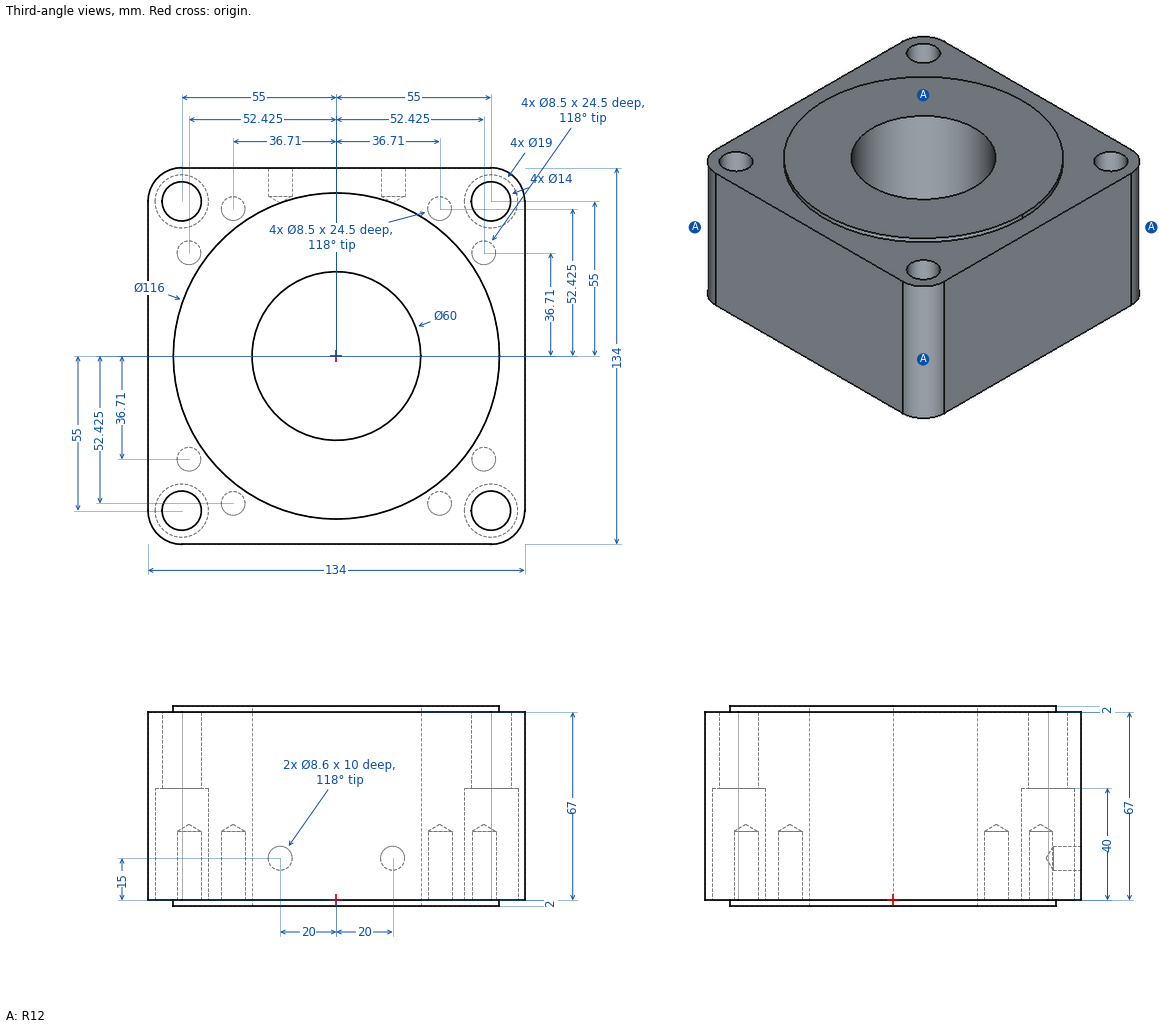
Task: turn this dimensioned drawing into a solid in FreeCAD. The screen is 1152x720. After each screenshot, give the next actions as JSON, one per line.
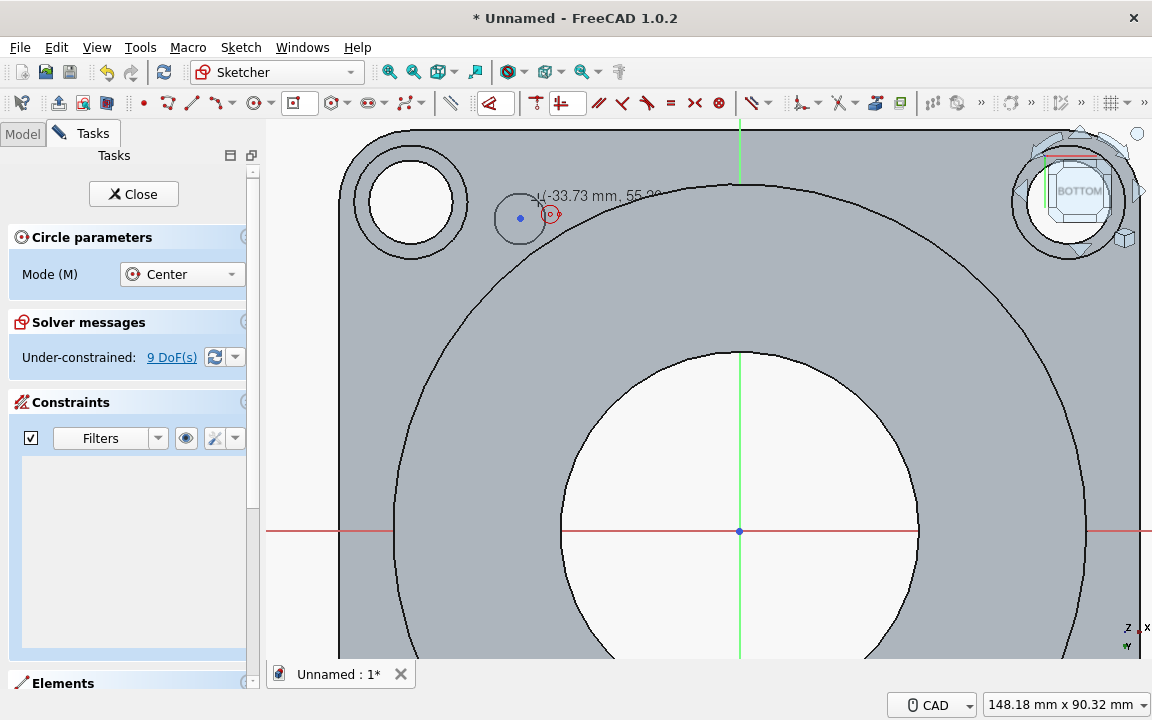
{"action": "left_click", "coordinate": [959, 218]}
{"action": "left_click", "coordinate": [977, 200]}
{"action": "key", "text": "Escape"}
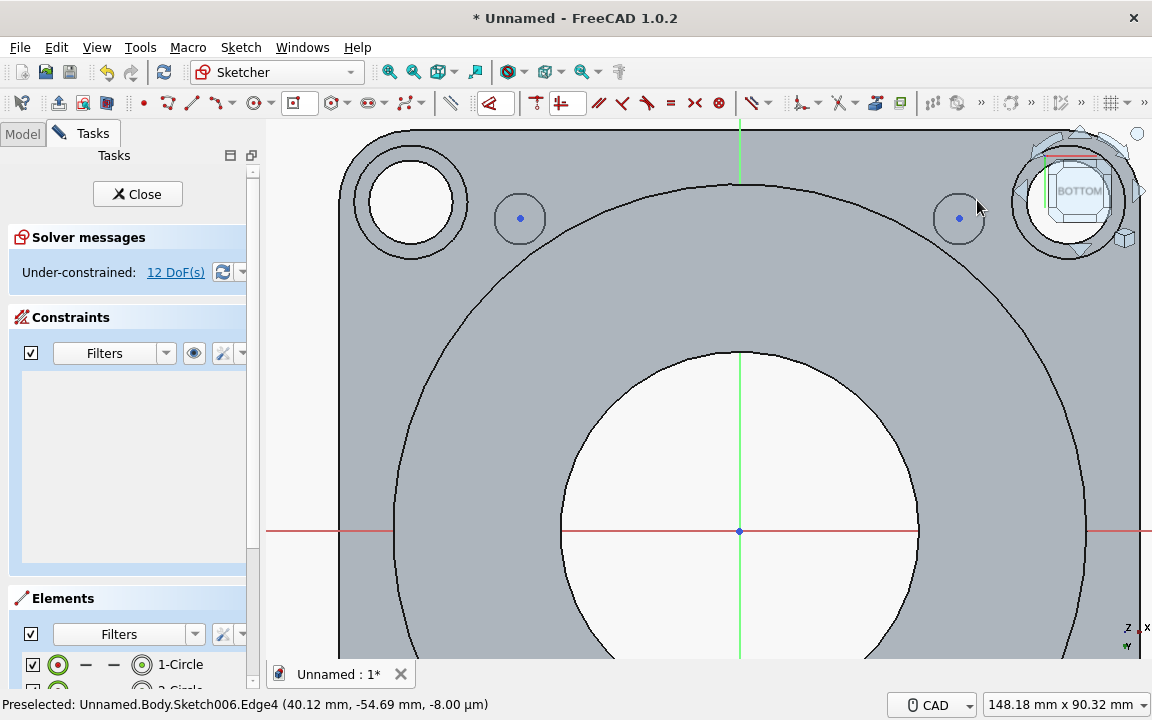
{"action": "scroll", "coordinate": [520, 216], "scroll_direction": "down", "scroll_amount": 3}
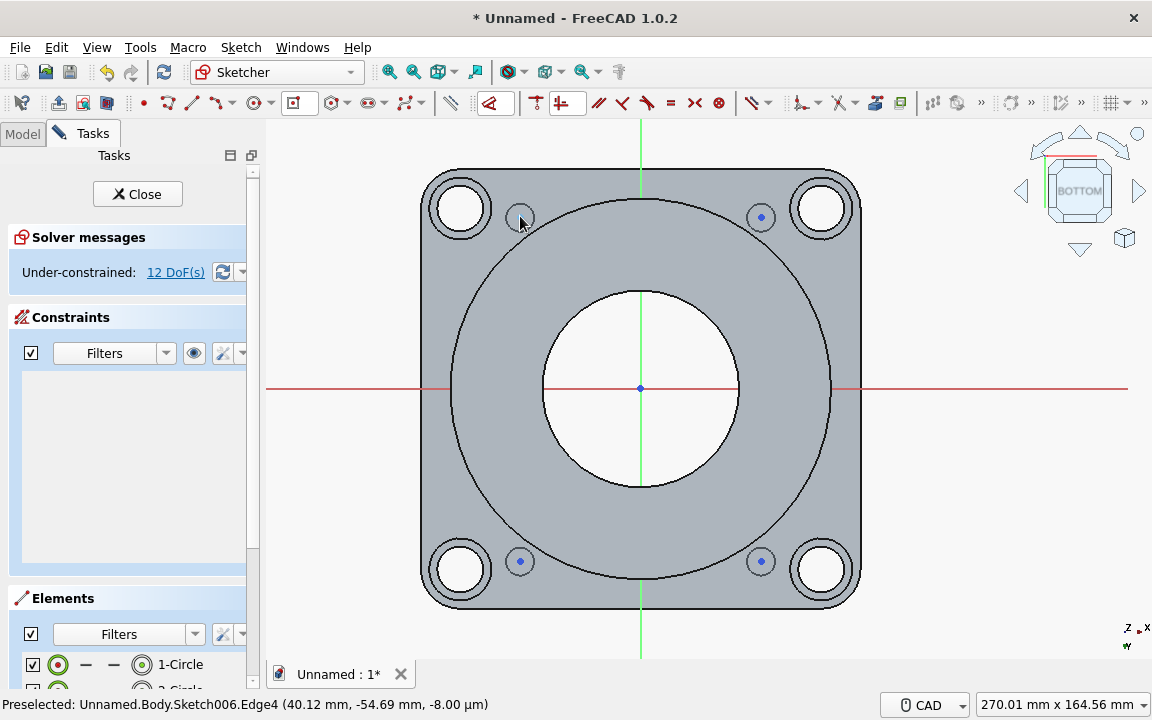
{"action": "left_click", "coordinate": [771, 552]}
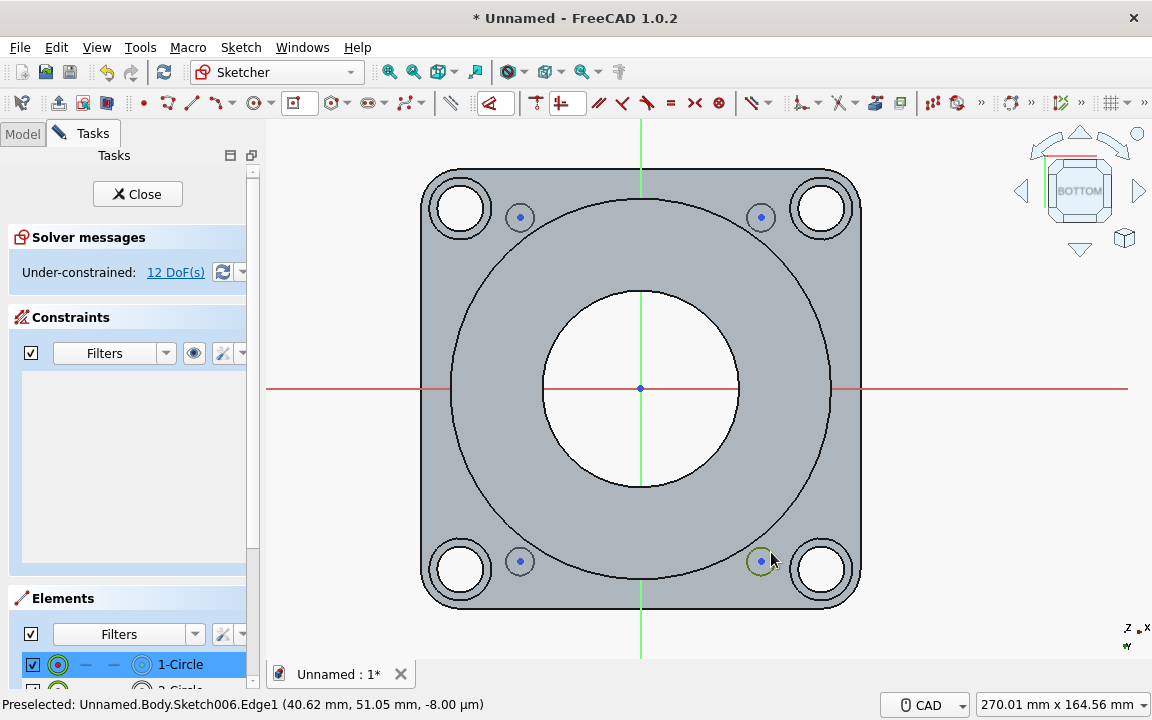
{"action": "left_click", "coordinate": [530, 552]}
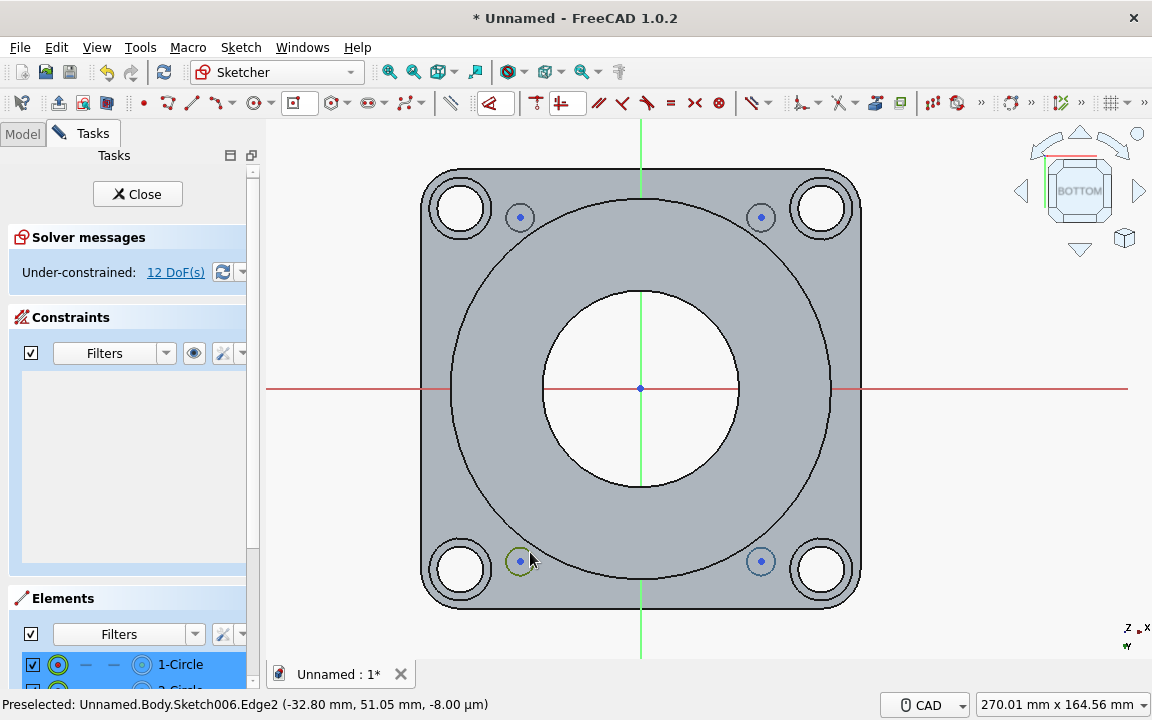
{"action": "left_click", "coordinate": [530, 208]}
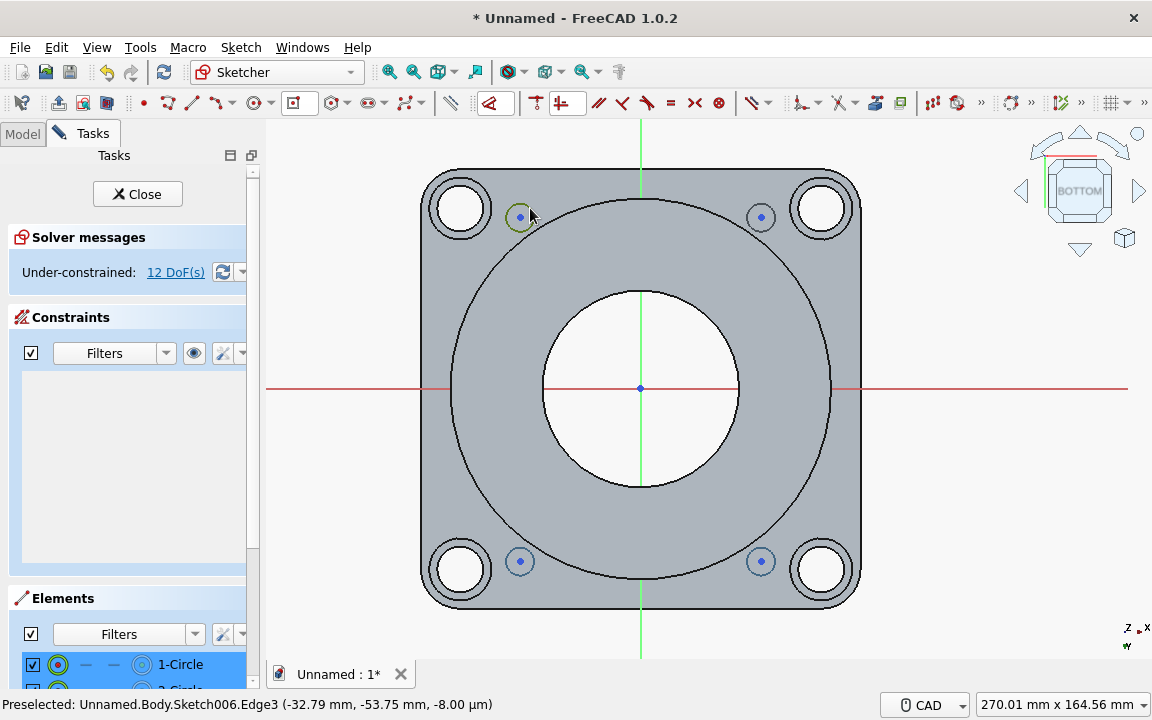
{"action": "left_click", "coordinate": [771, 208]}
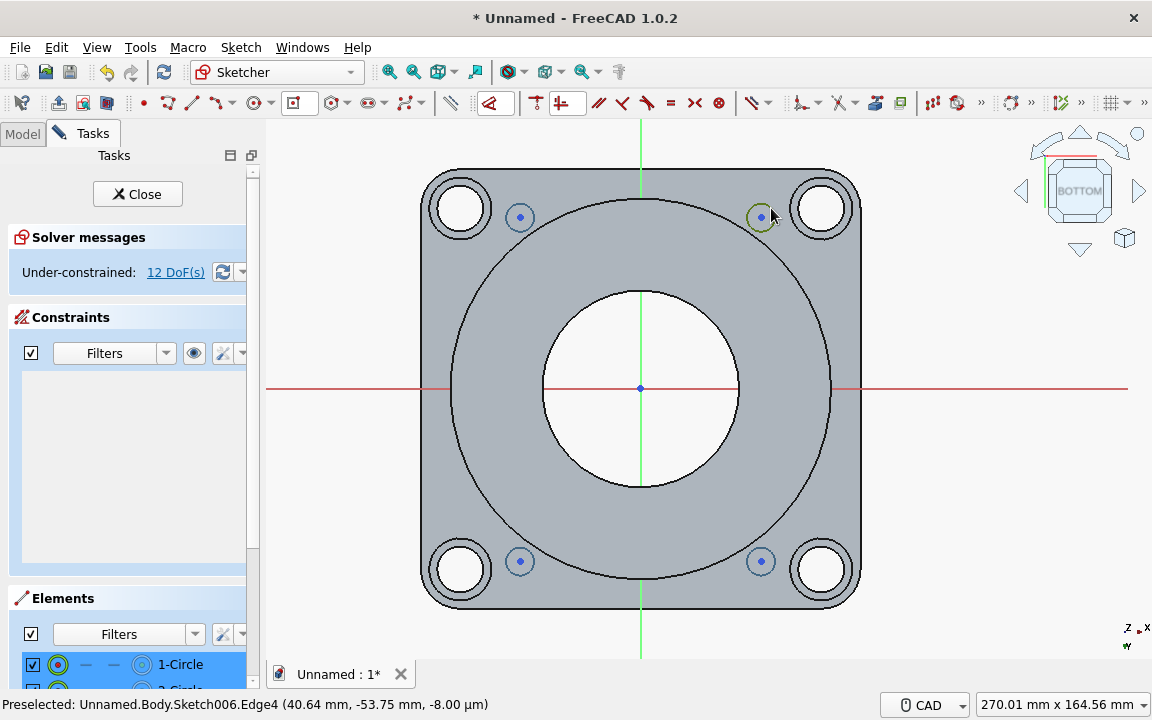
{"action": "left_click", "coordinate": [672, 104]}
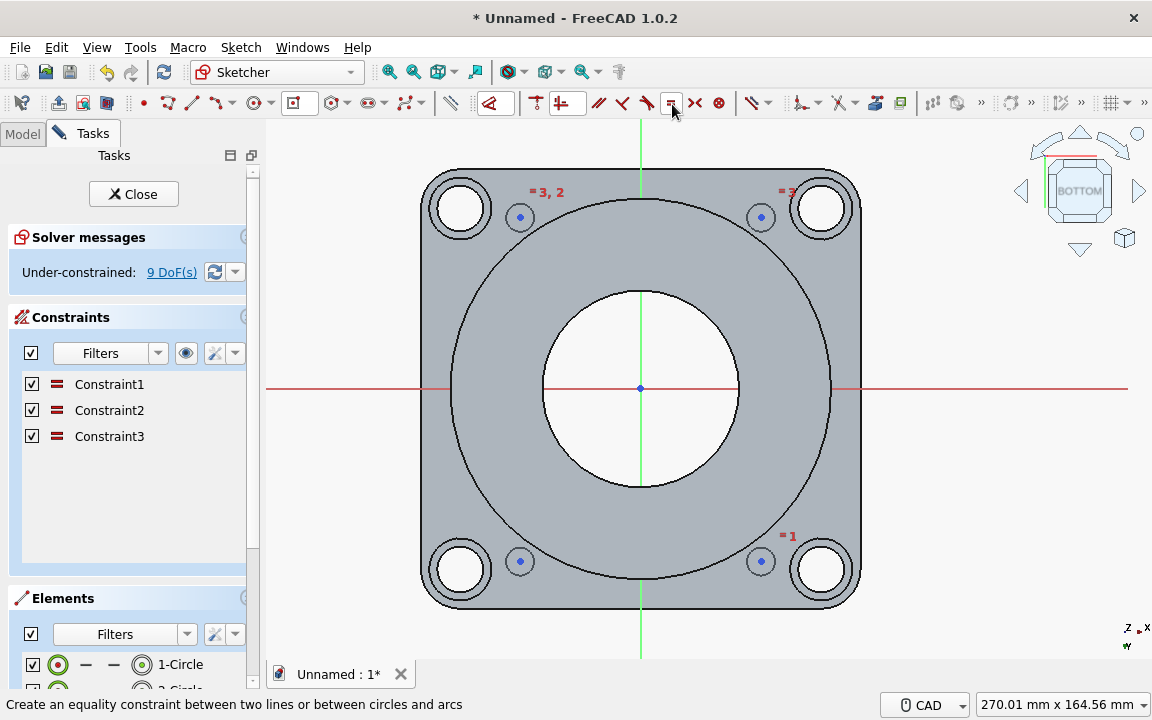
{"action": "left_click", "coordinate": [761, 562]}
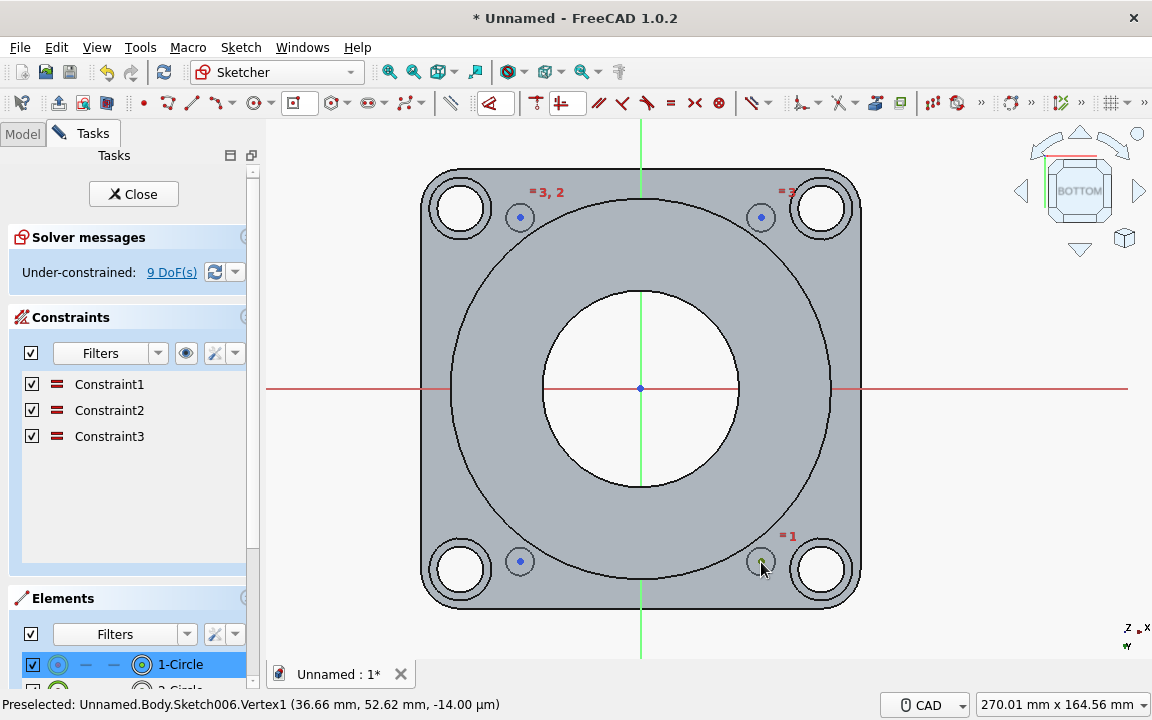
{"action": "left_click", "coordinate": [520, 562]}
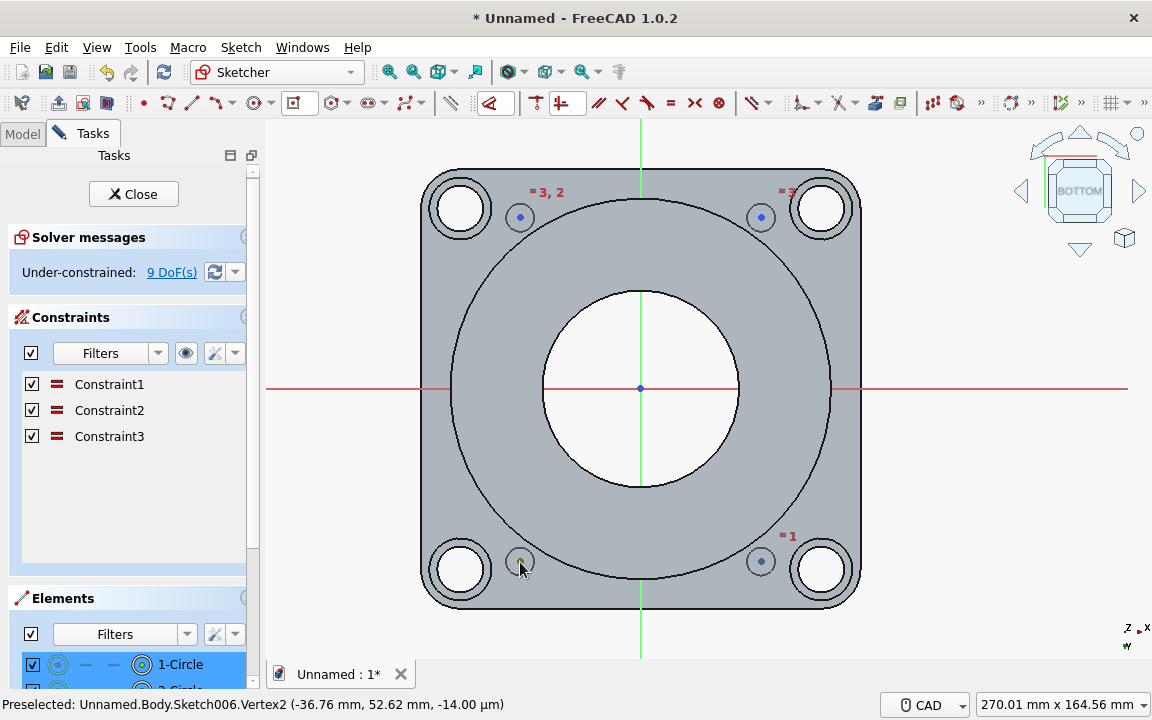
{"action": "key", "text": "h"}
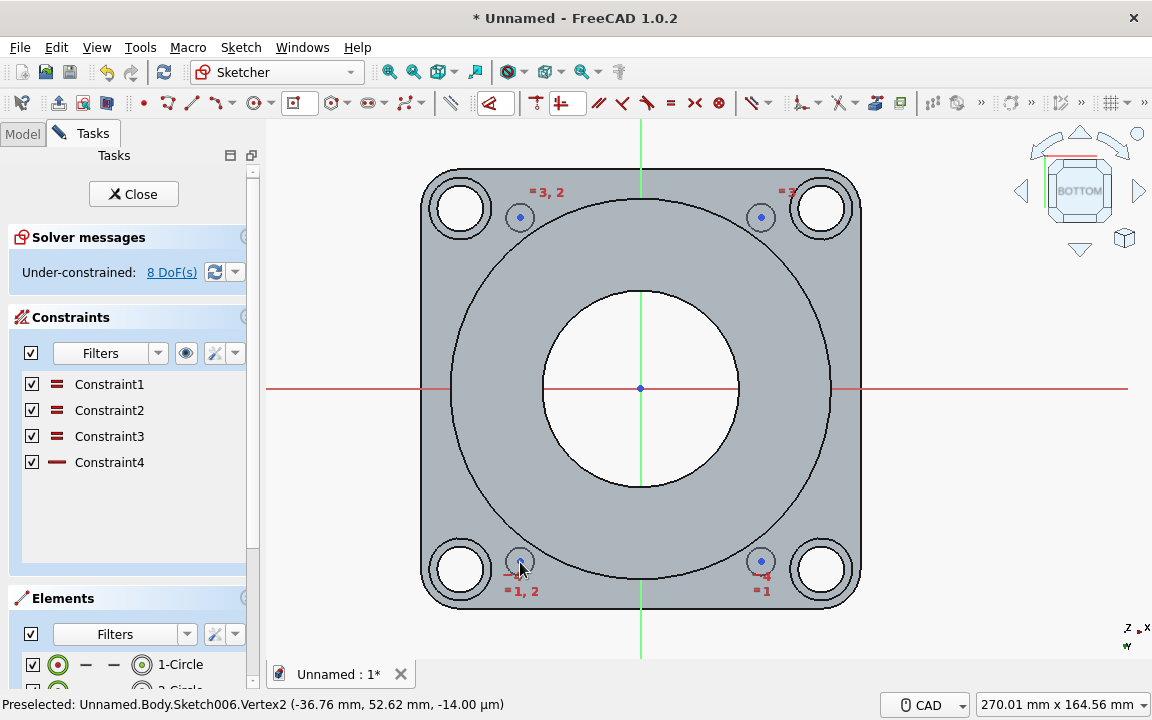
{"action": "left_click", "coordinate": [520, 562]}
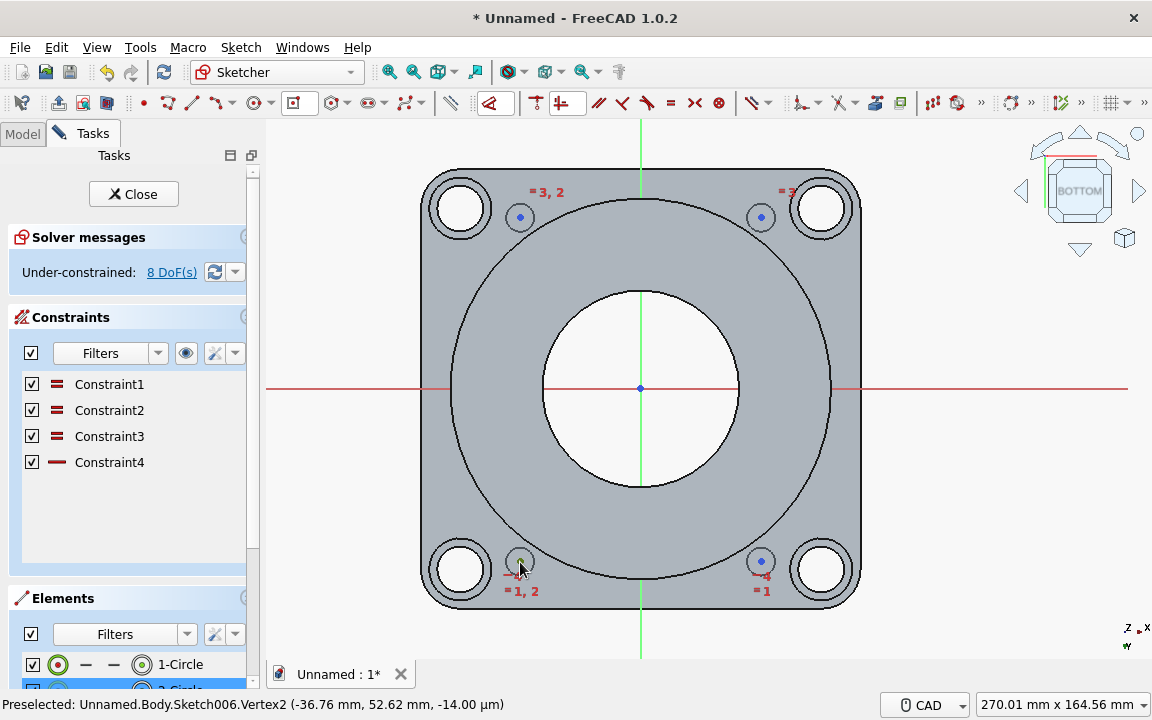
{"action": "left_click", "coordinate": [520, 218]}